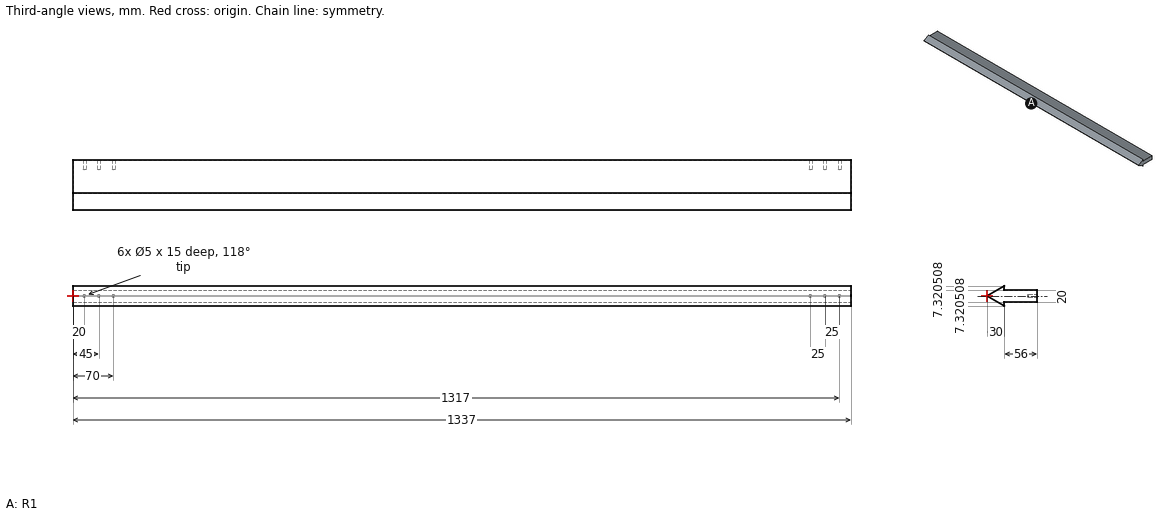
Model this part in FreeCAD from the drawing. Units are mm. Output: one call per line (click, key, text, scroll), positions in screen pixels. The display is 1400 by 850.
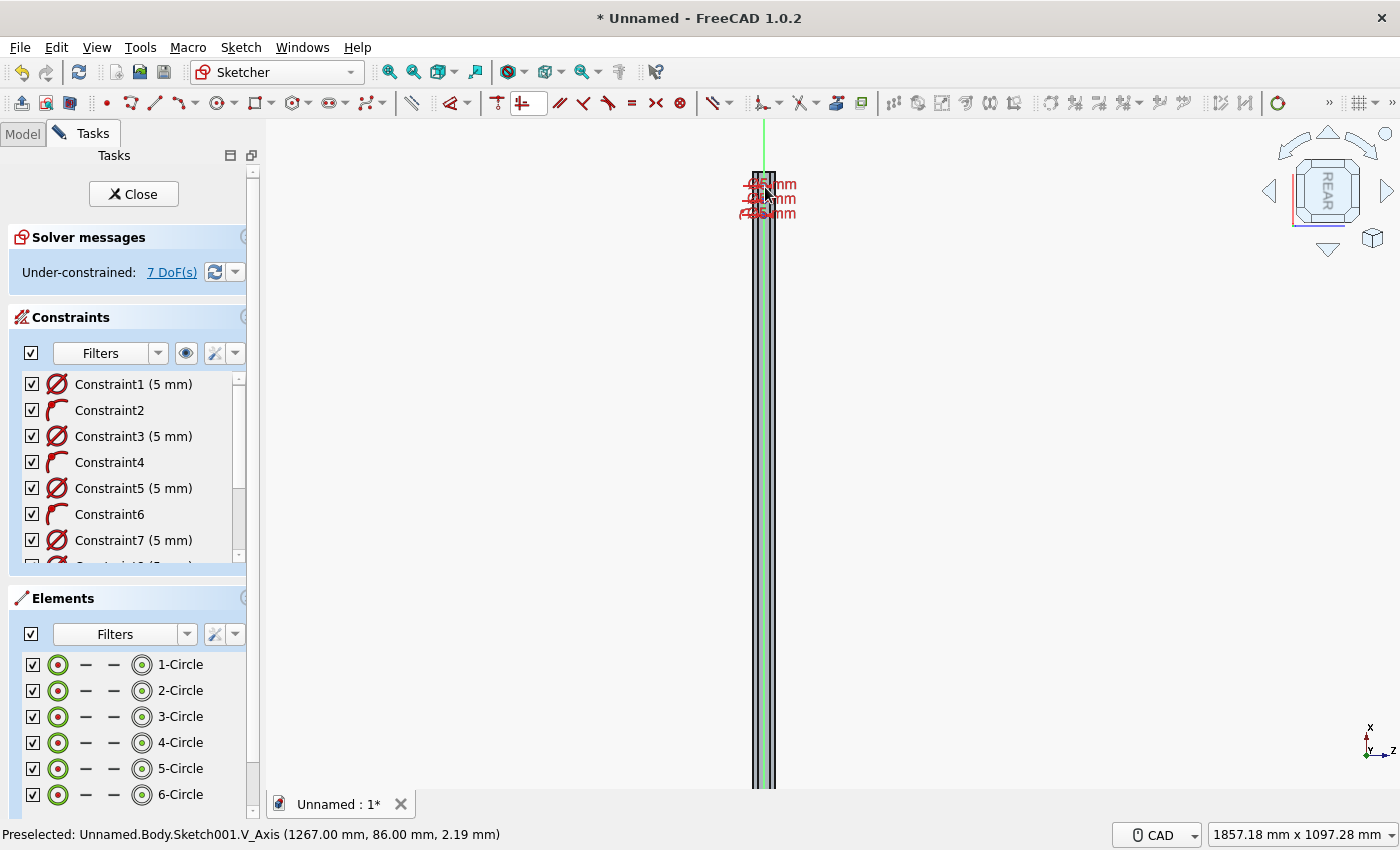
click(765, 186)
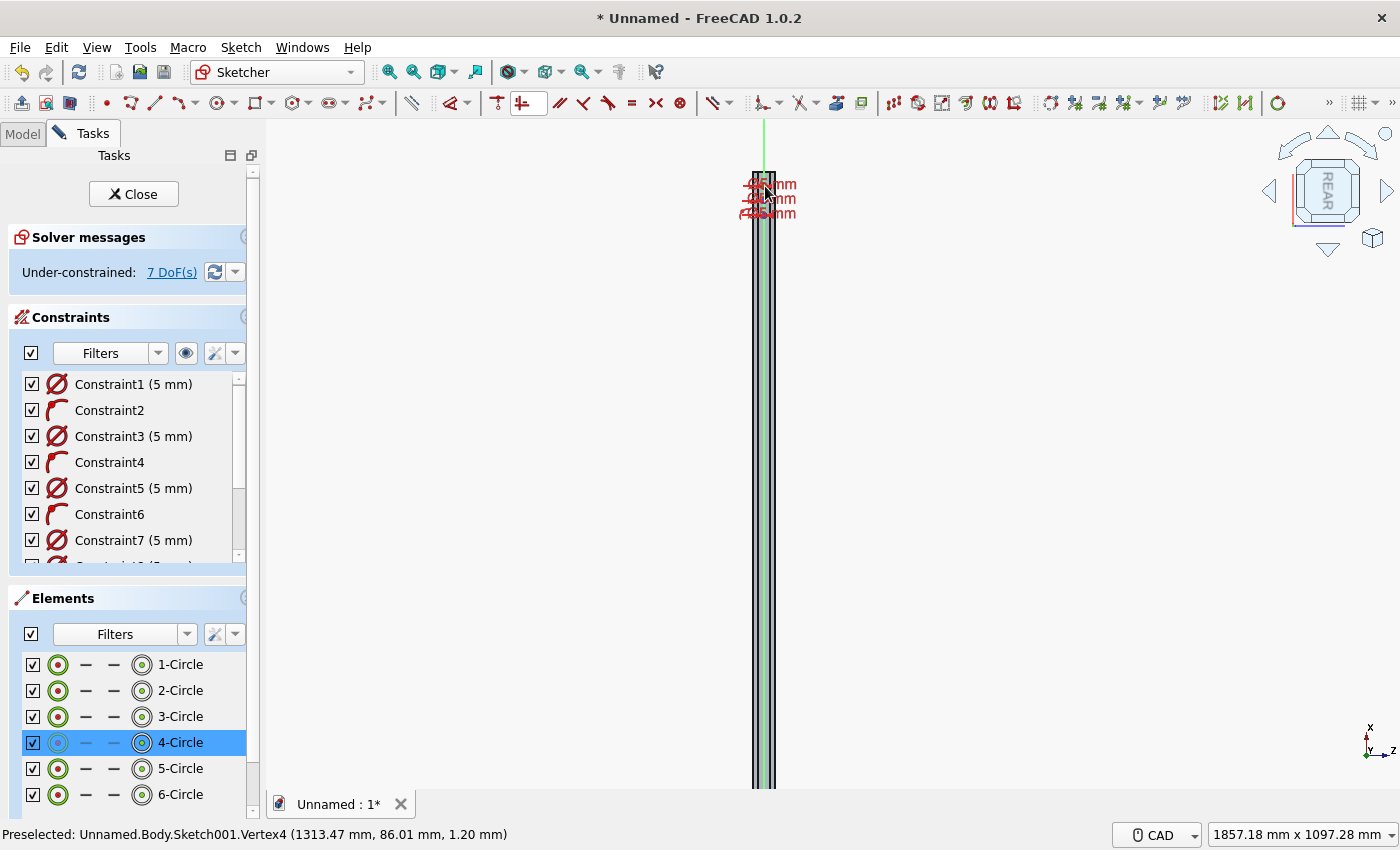
click(764, 717)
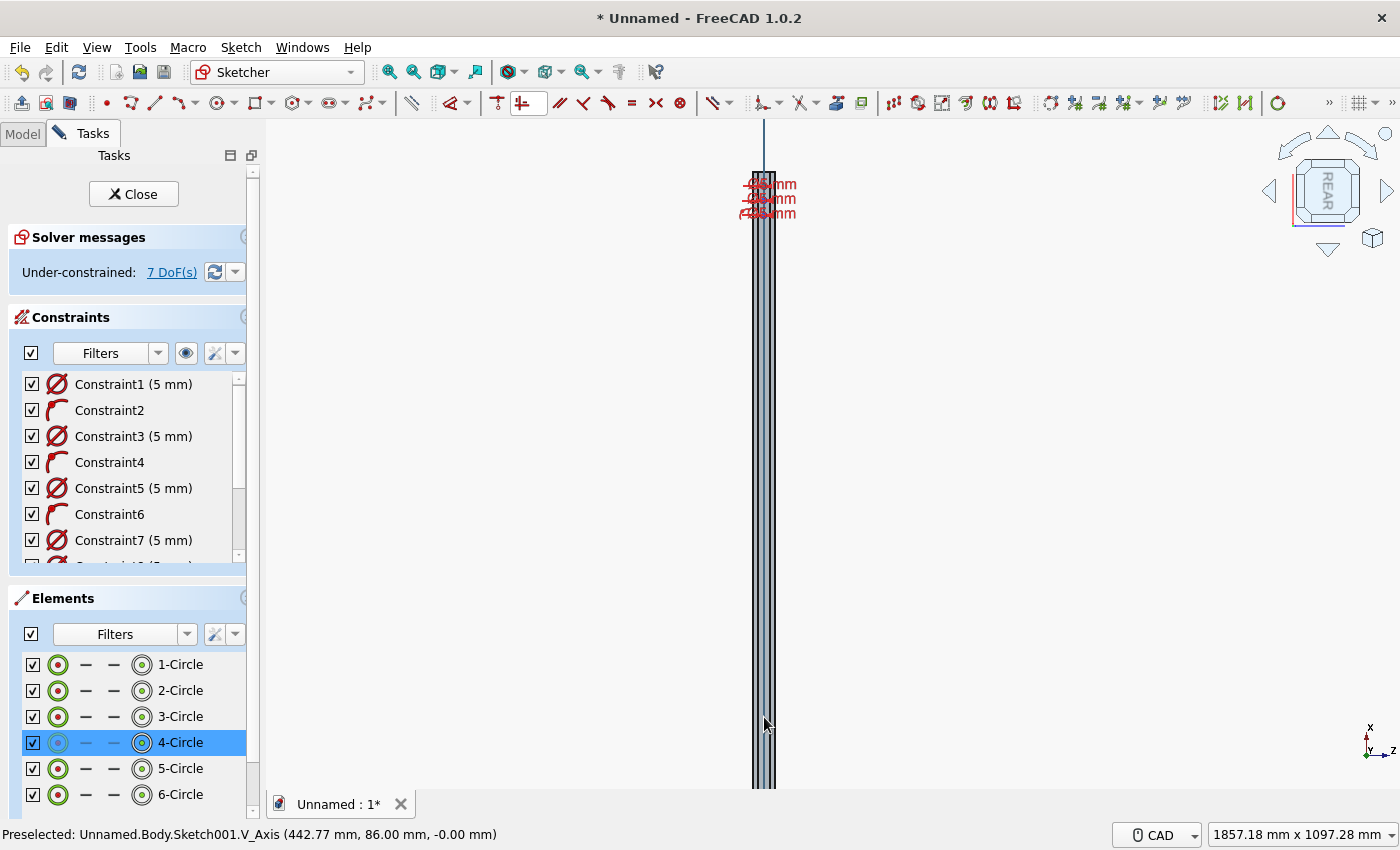
click(498, 104)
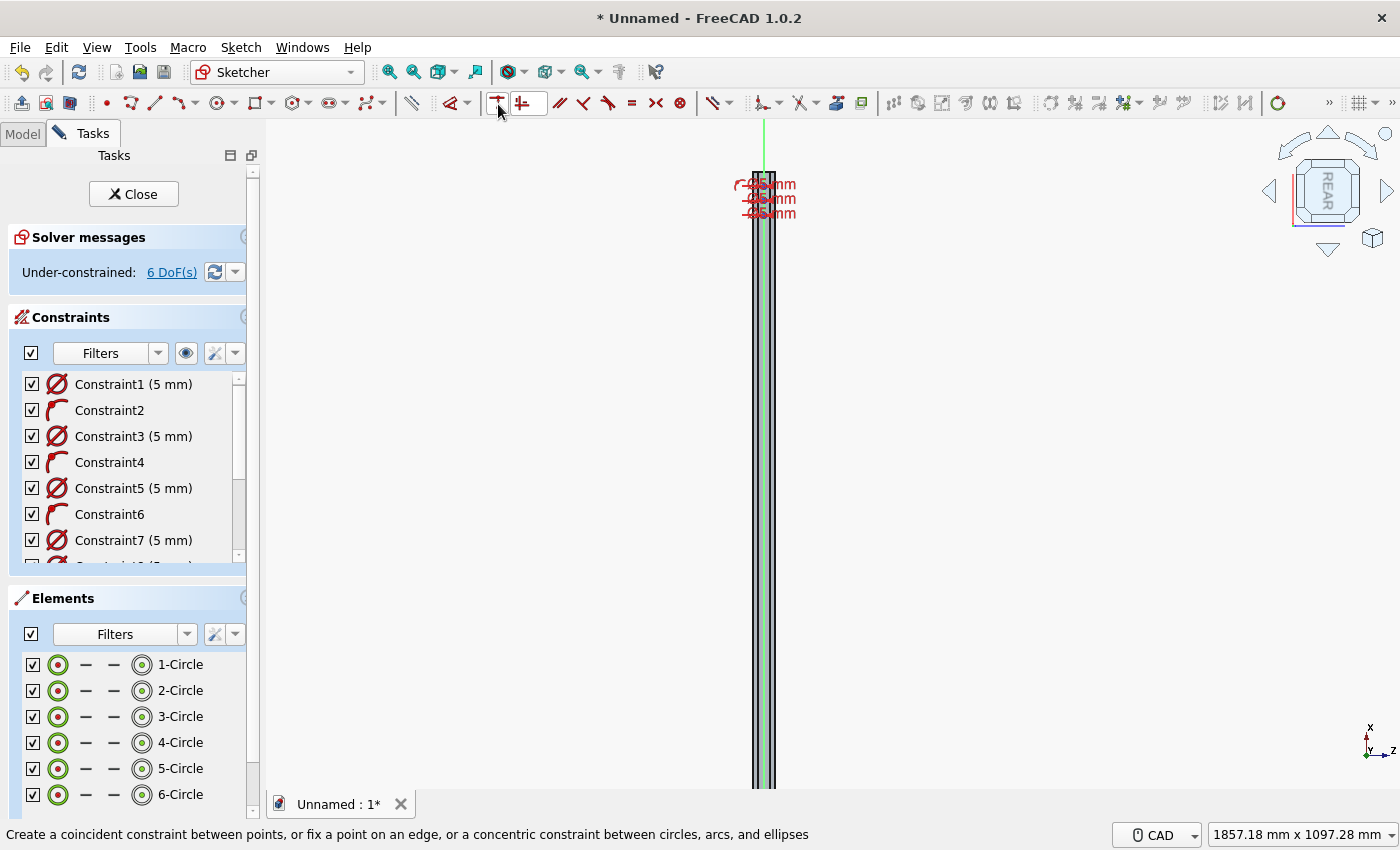
click(450, 104)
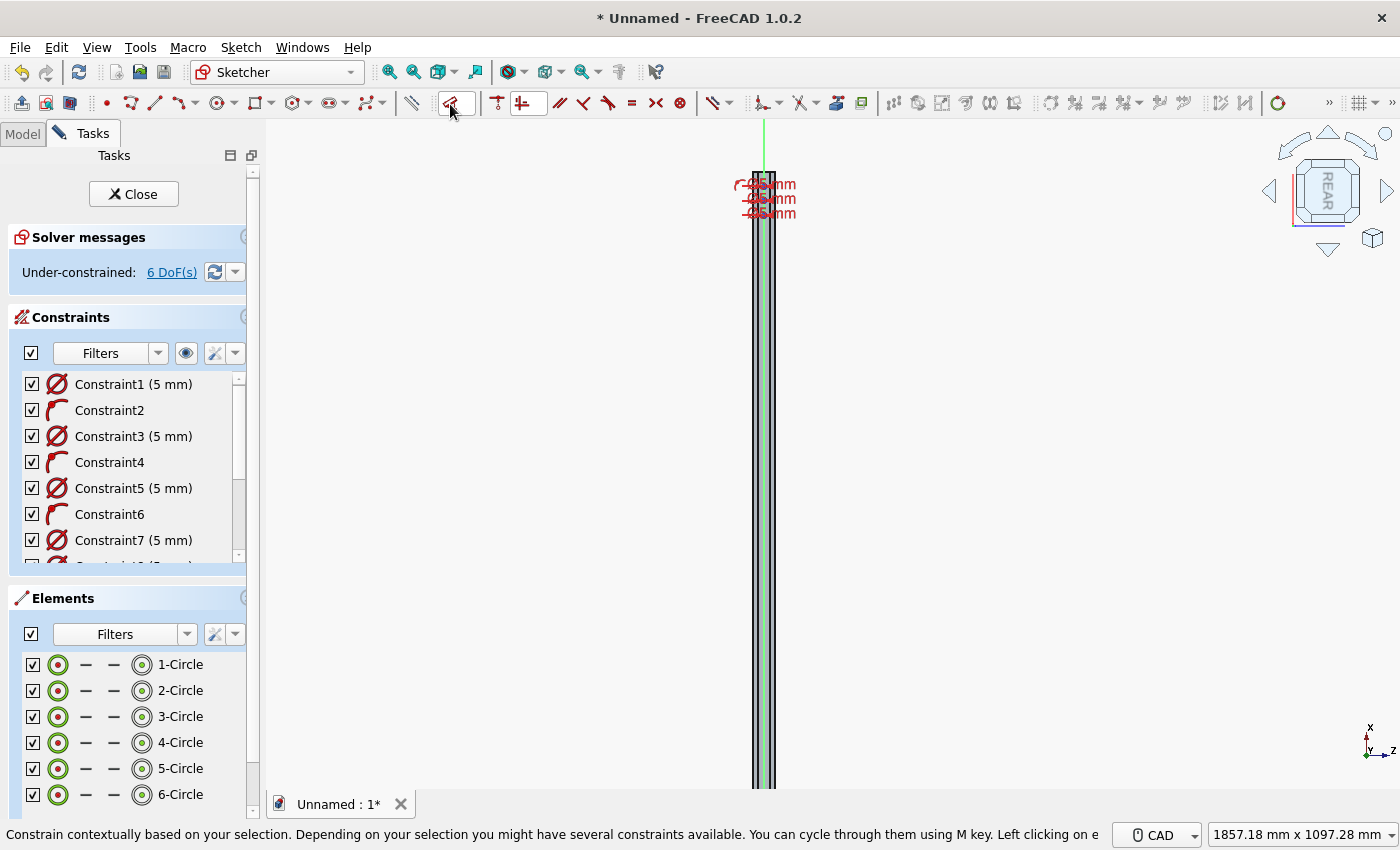
scroll(765, 294, down, 3)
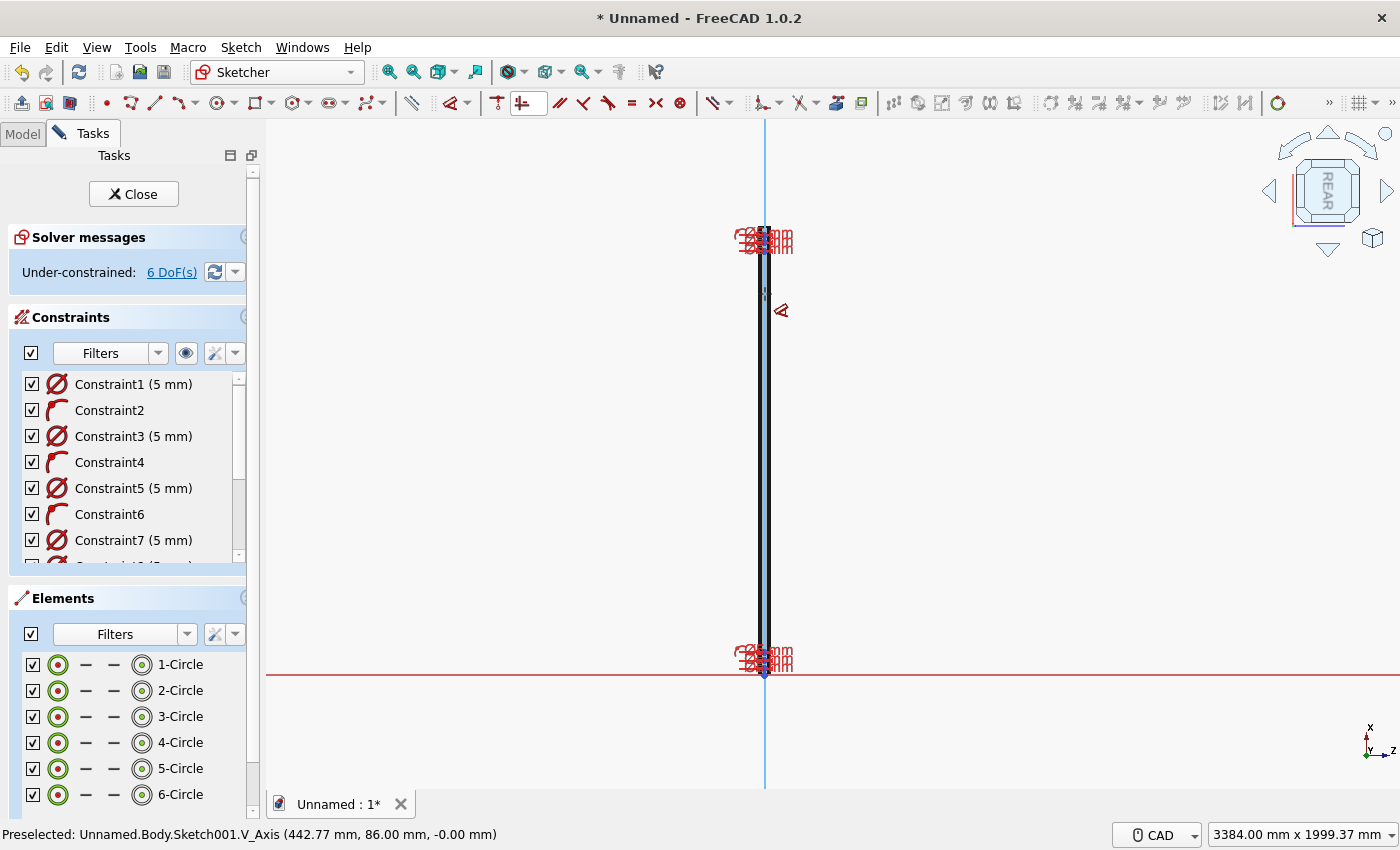
scroll(765, 669, up, 9)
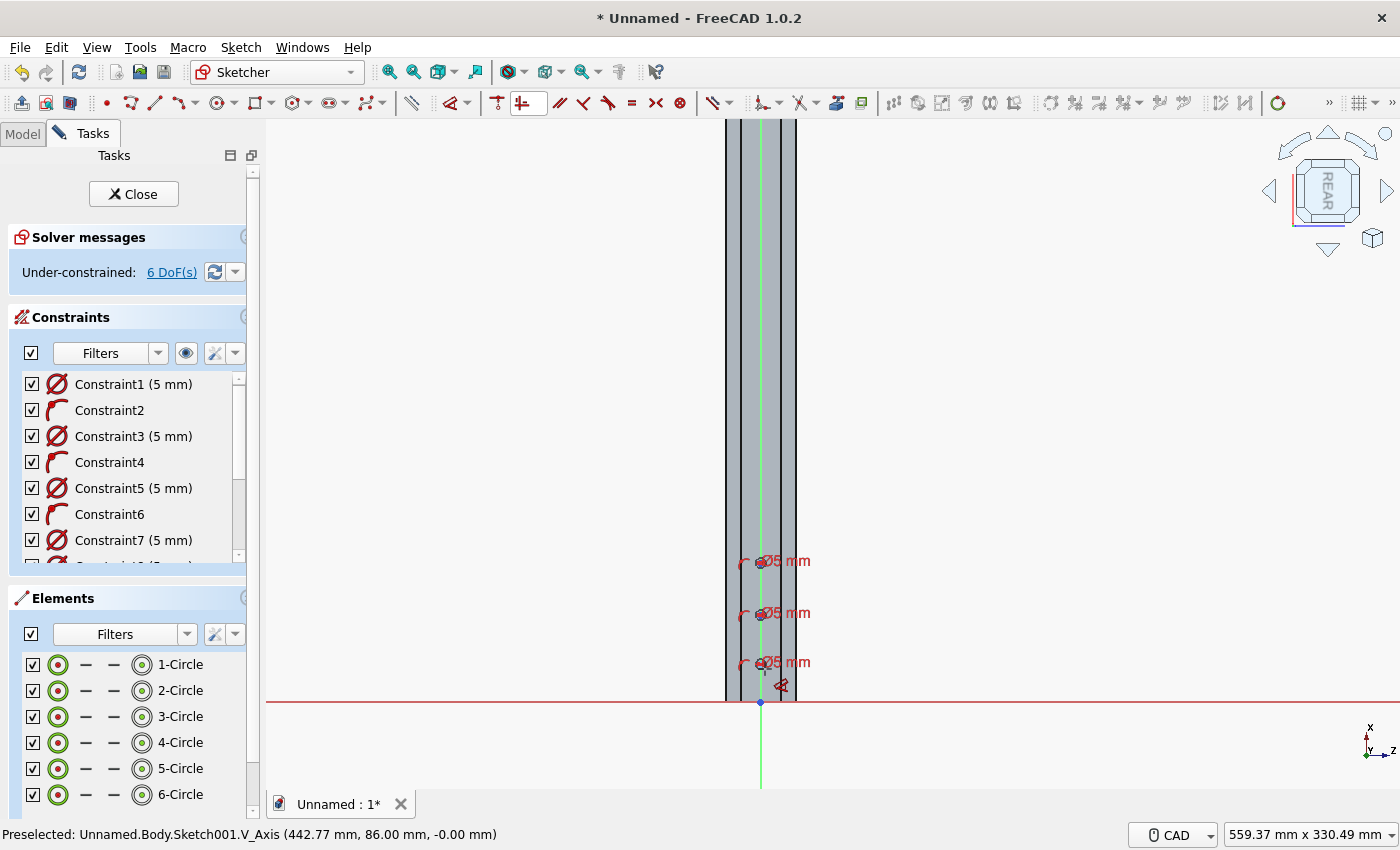
click(761, 664)
click(795, 683)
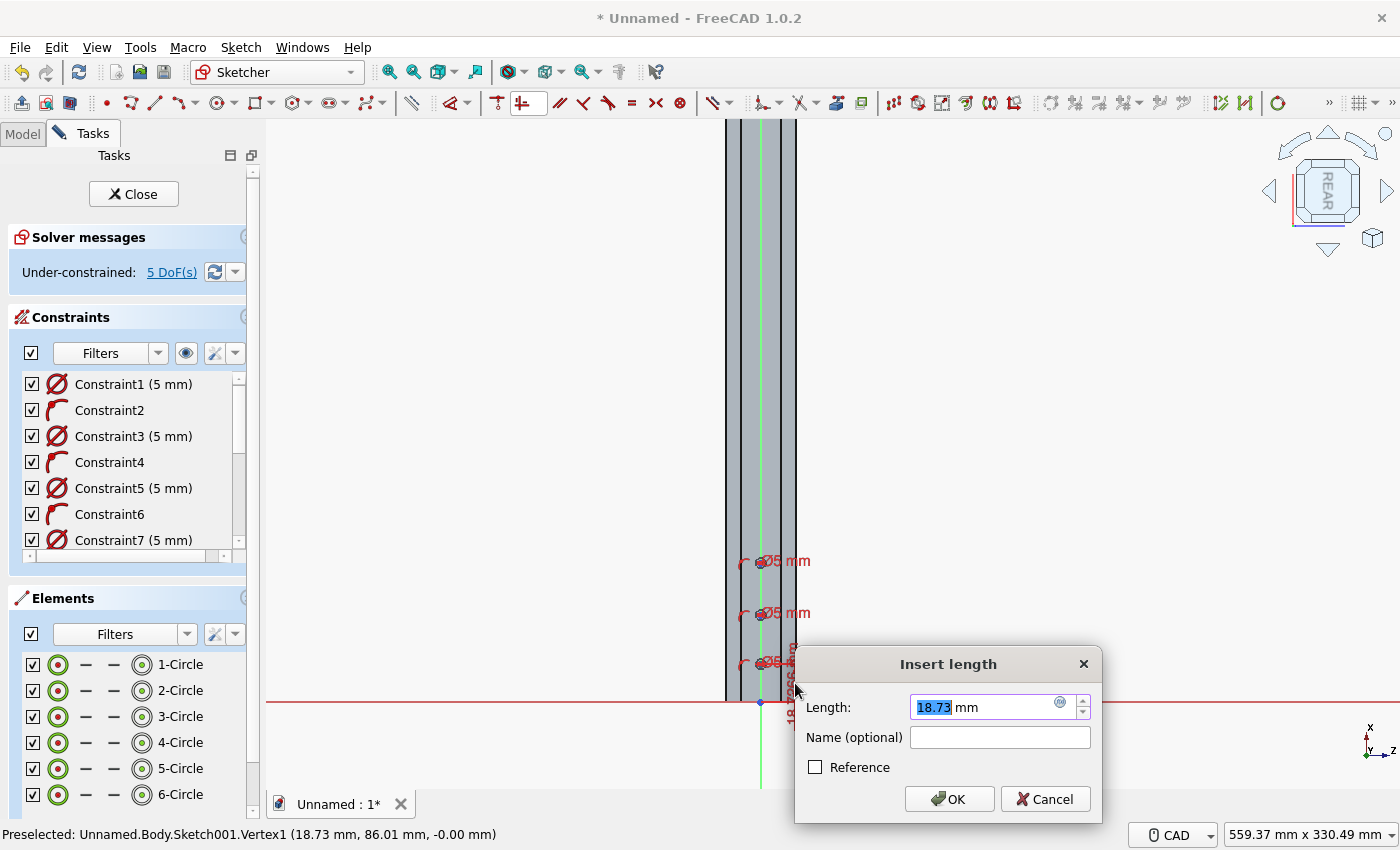
text(20)
key(Return)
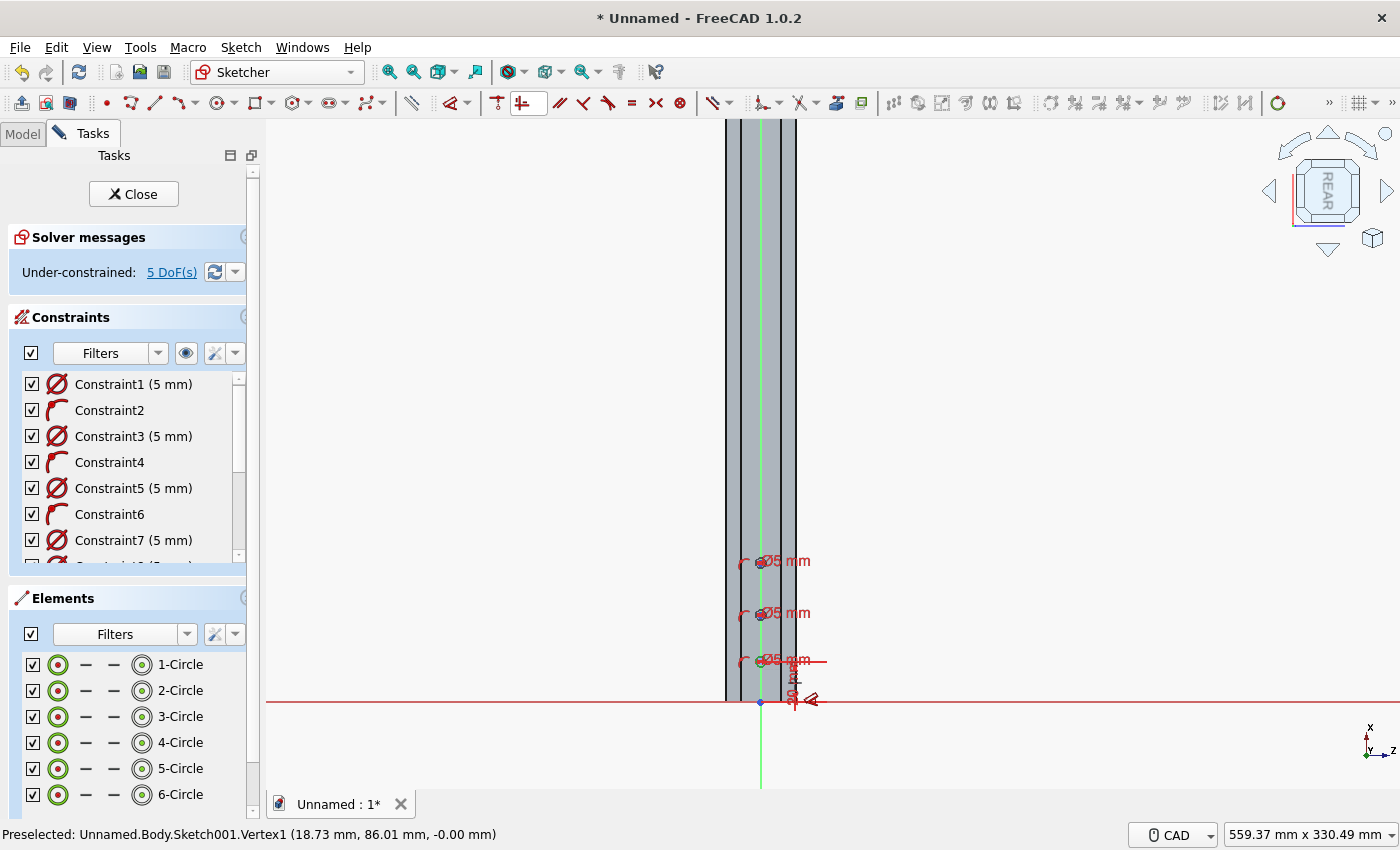
click(761, 615)
click(795, 659)